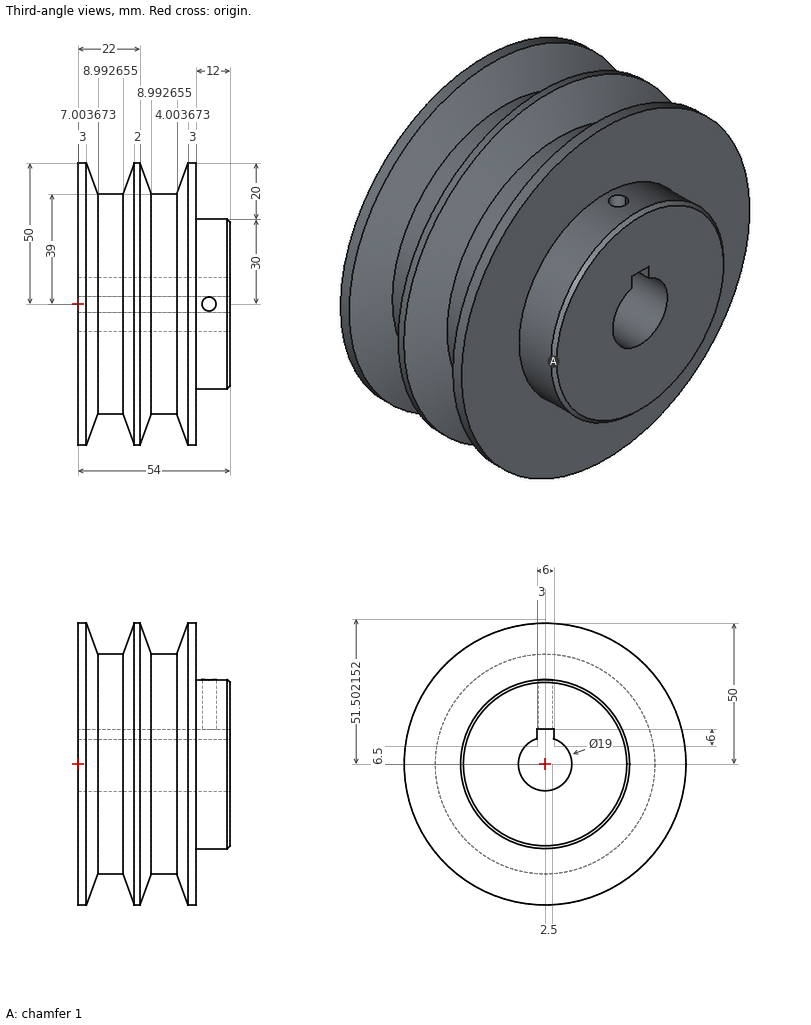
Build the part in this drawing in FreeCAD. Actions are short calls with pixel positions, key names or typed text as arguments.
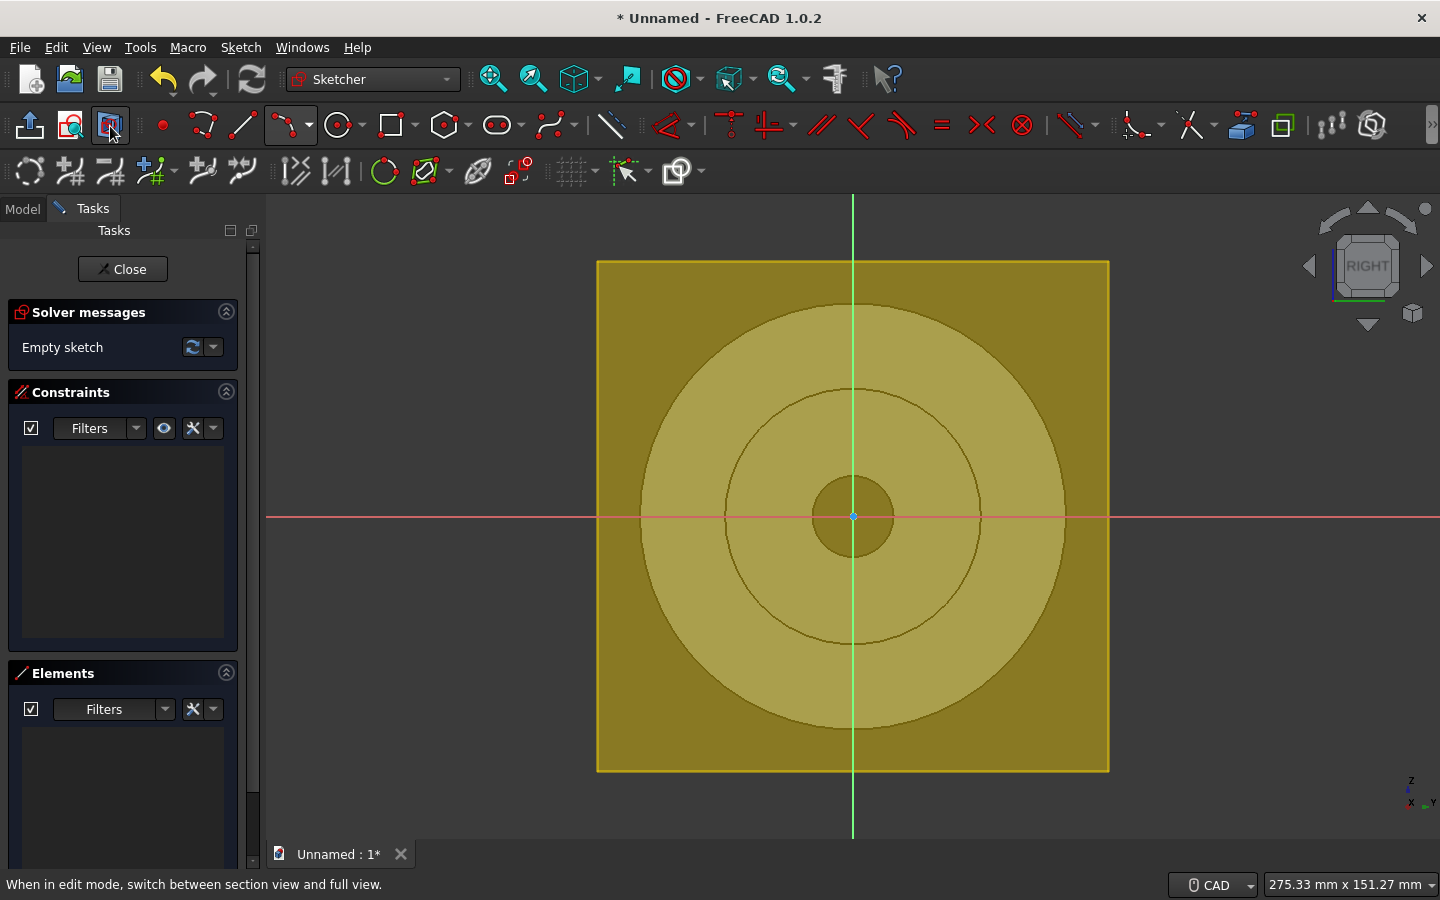
scroll(948, 273, up, 3)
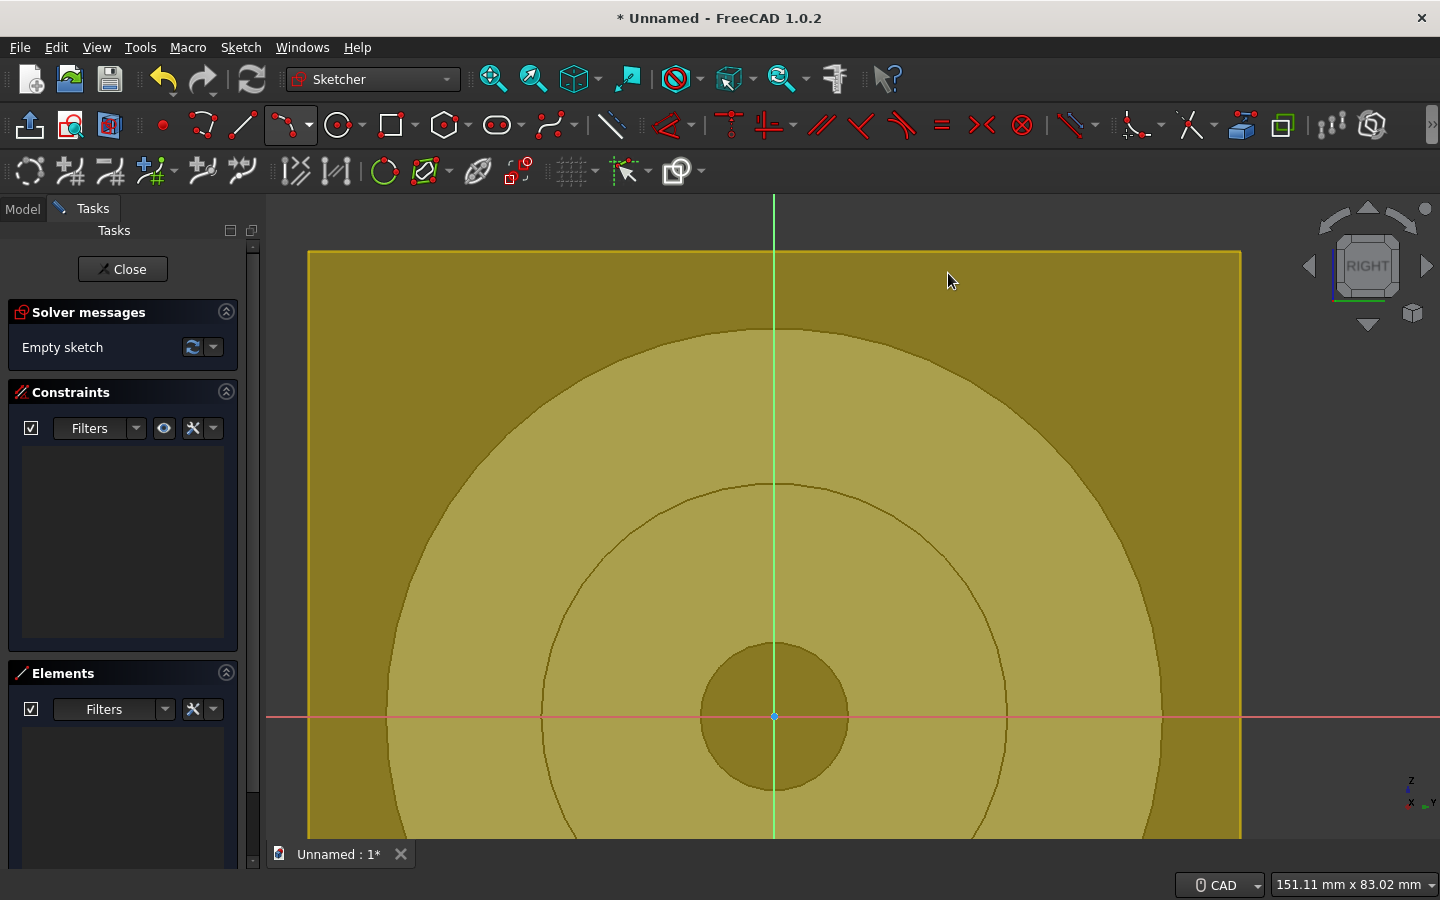
click(204, 126)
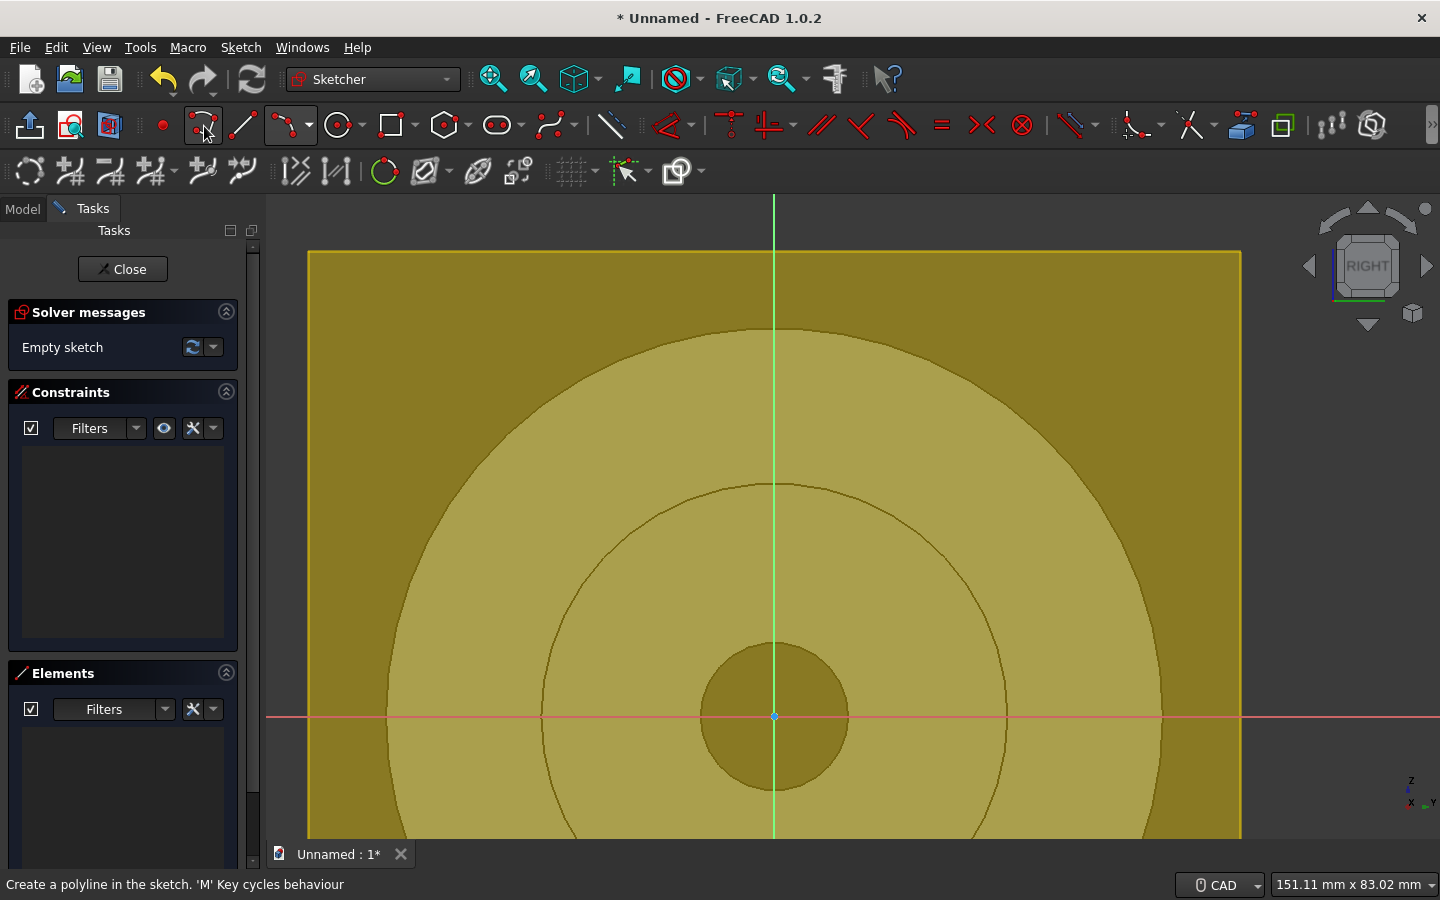
click(774, 717)
click(794, 708)
click(794, 328)
click(783, 316)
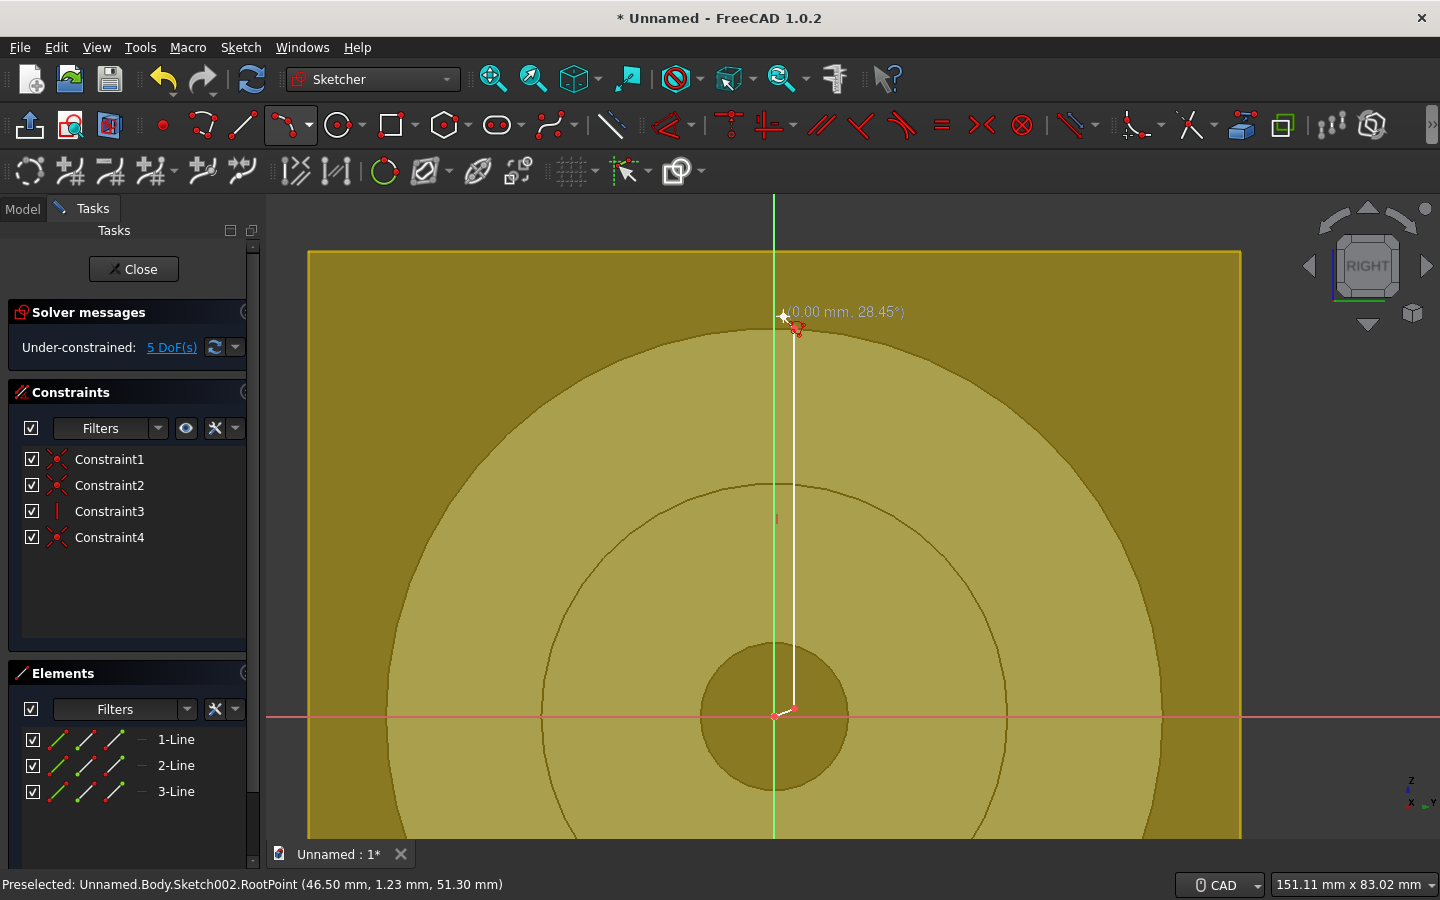
scroll(774, 717, up, 3)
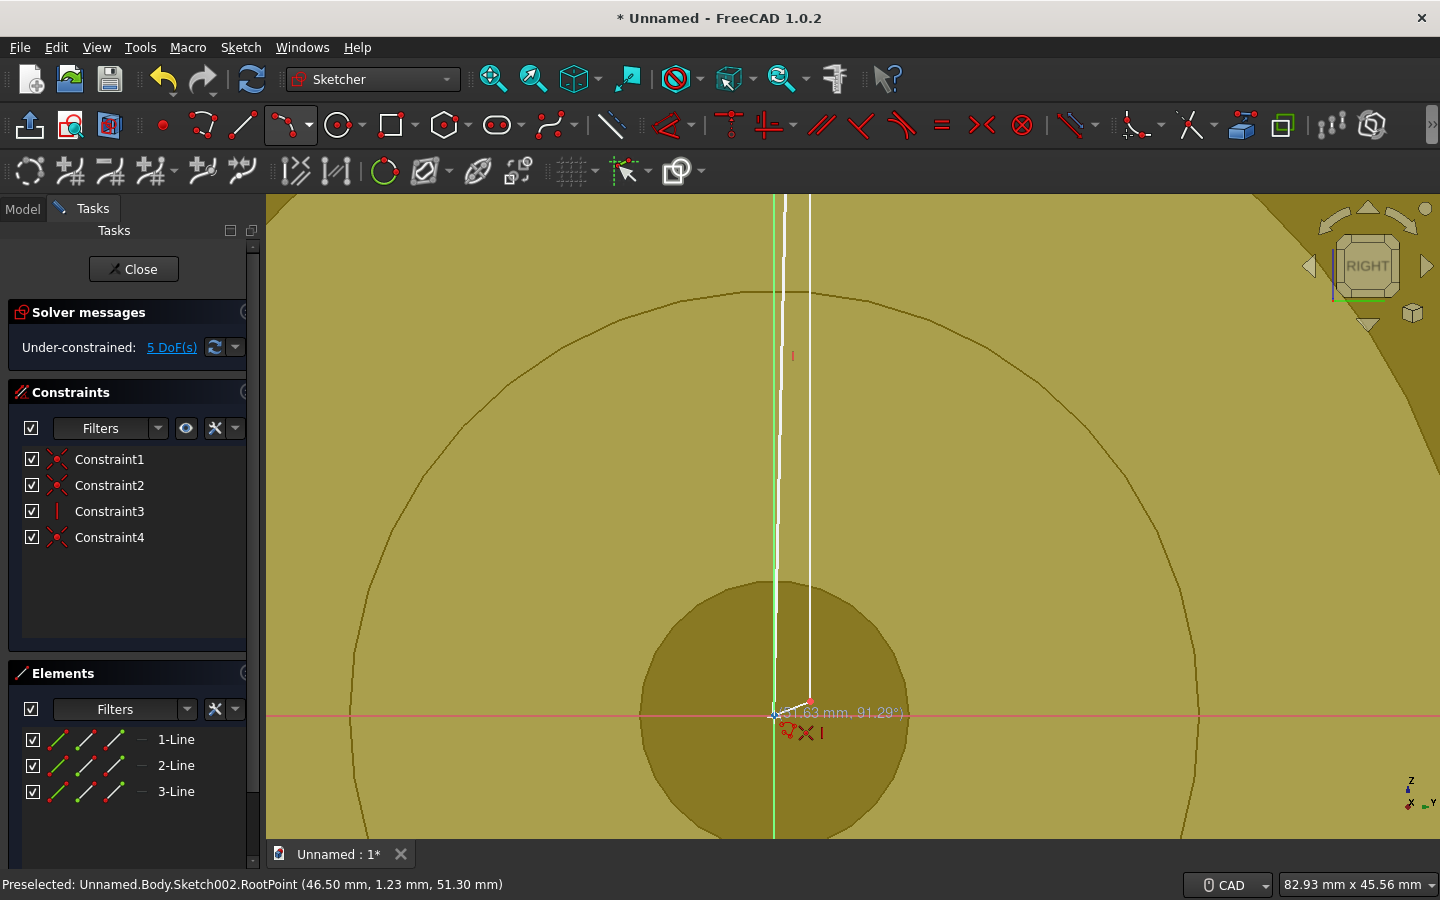
click(774, 716)
key(Escape)
key(Escape)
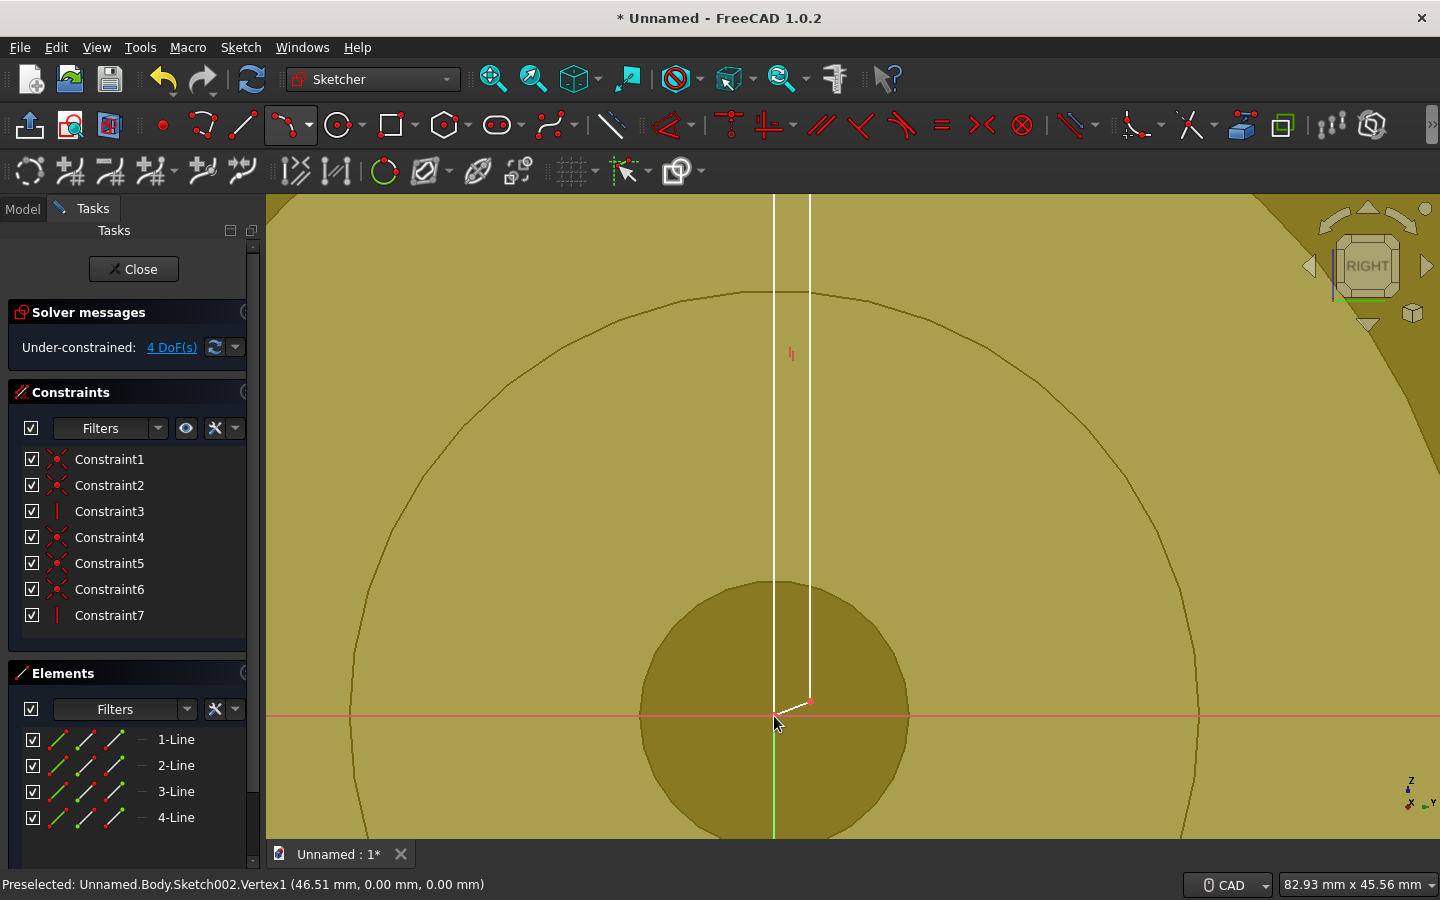
scroll(799, 706, up, 2)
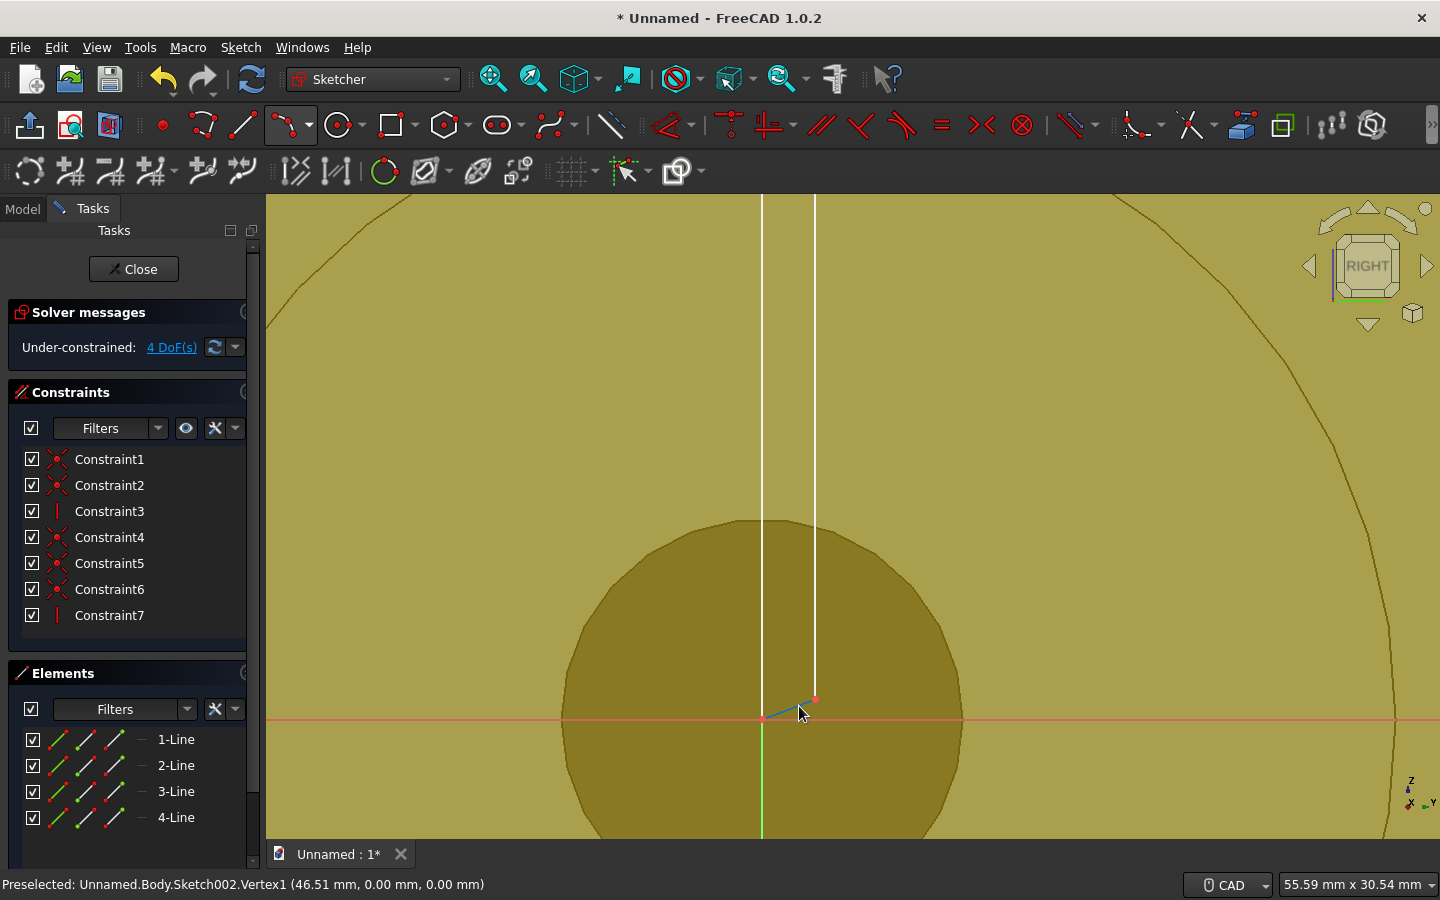
click(799, 705)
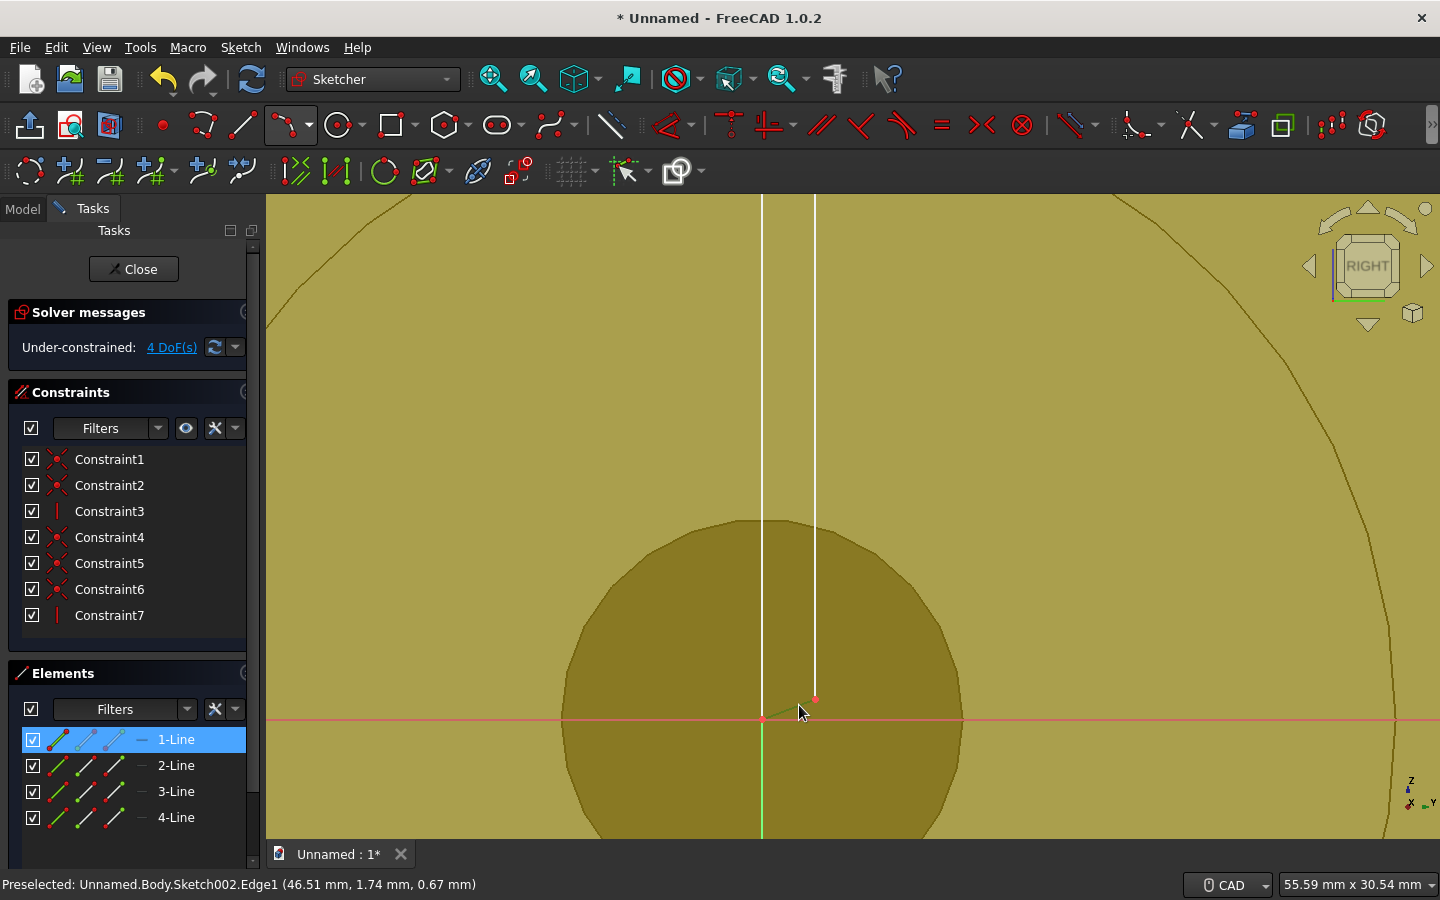
click(796, 126)